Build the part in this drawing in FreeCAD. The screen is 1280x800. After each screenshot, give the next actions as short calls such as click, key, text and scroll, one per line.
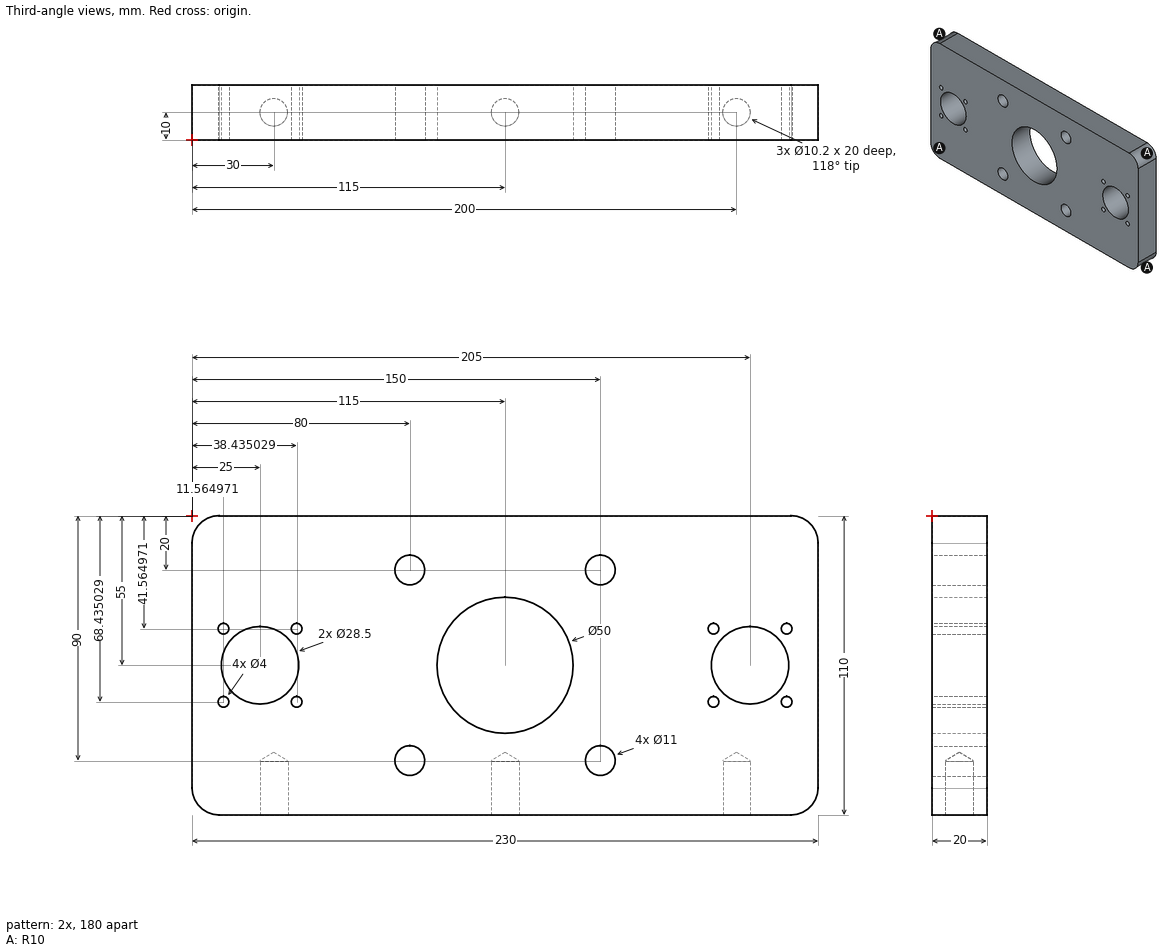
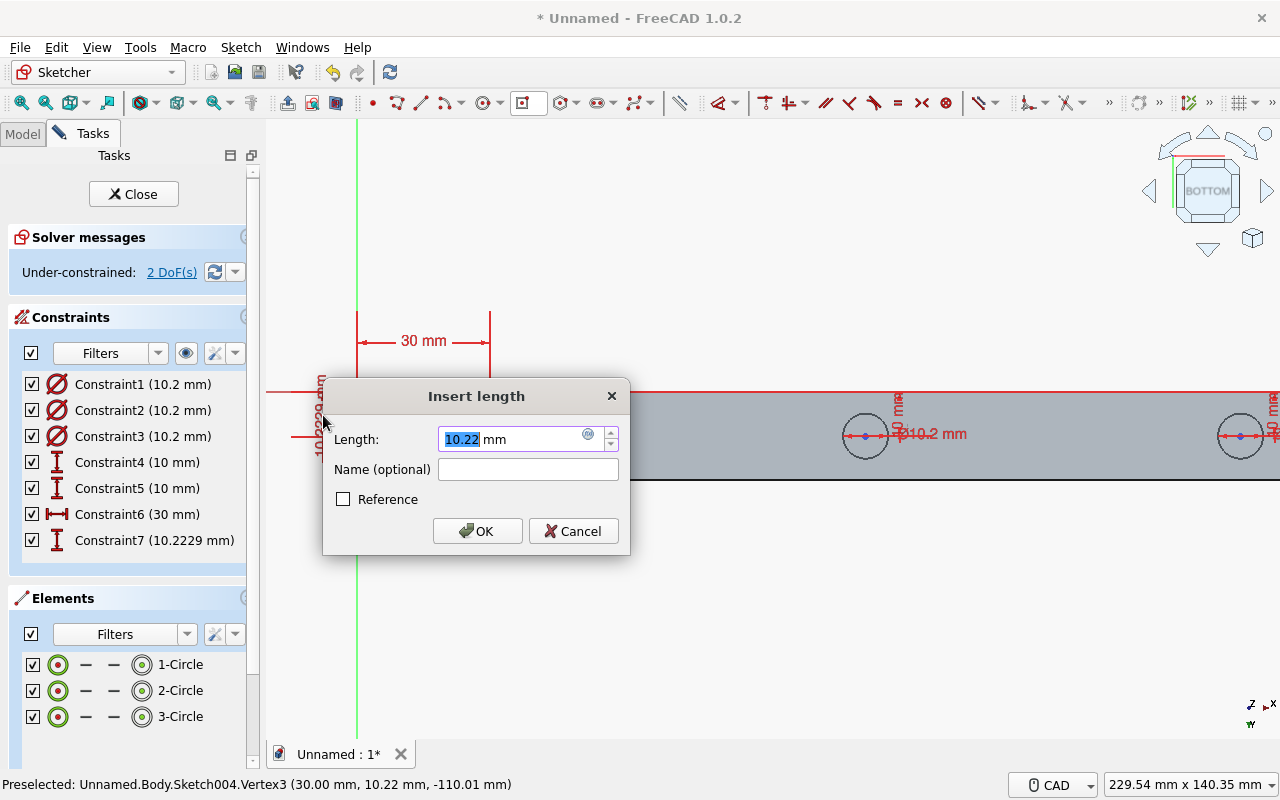
text(10)
key(Return)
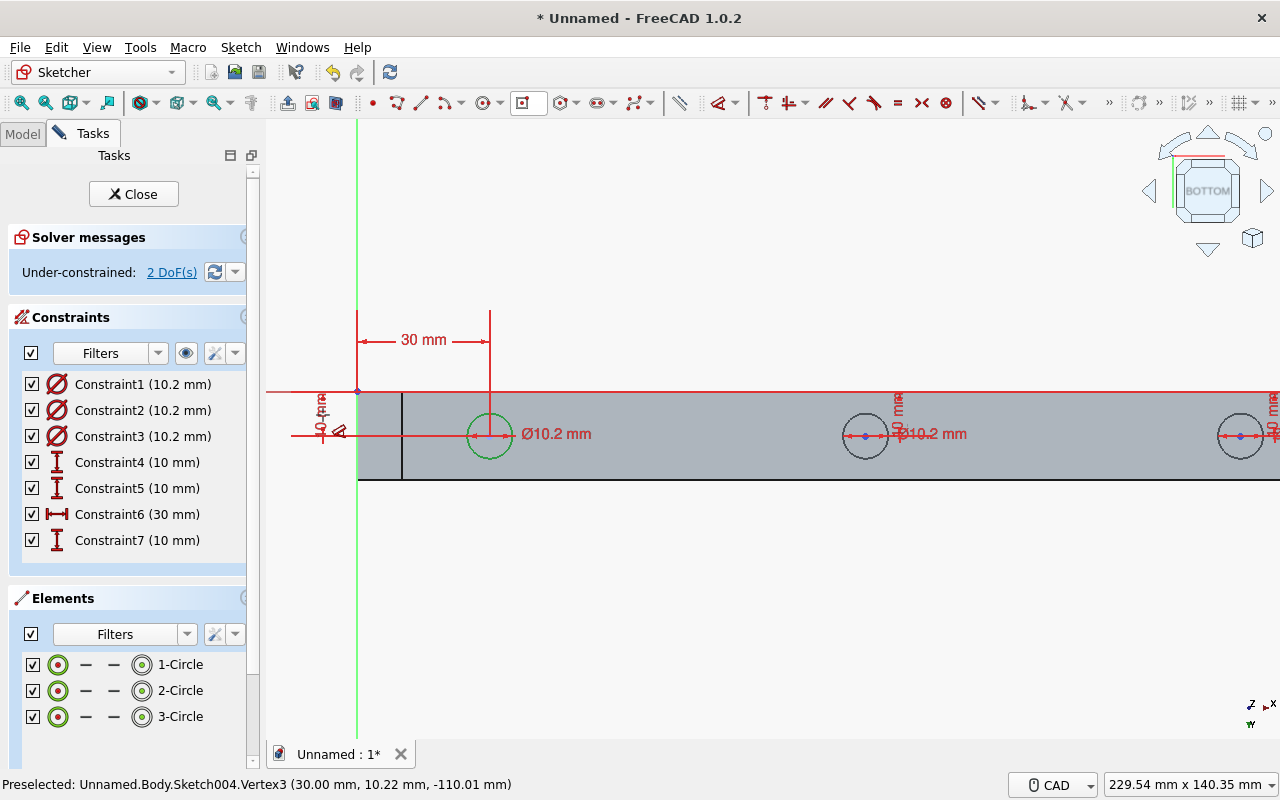
scroll(489, 437, down, 2)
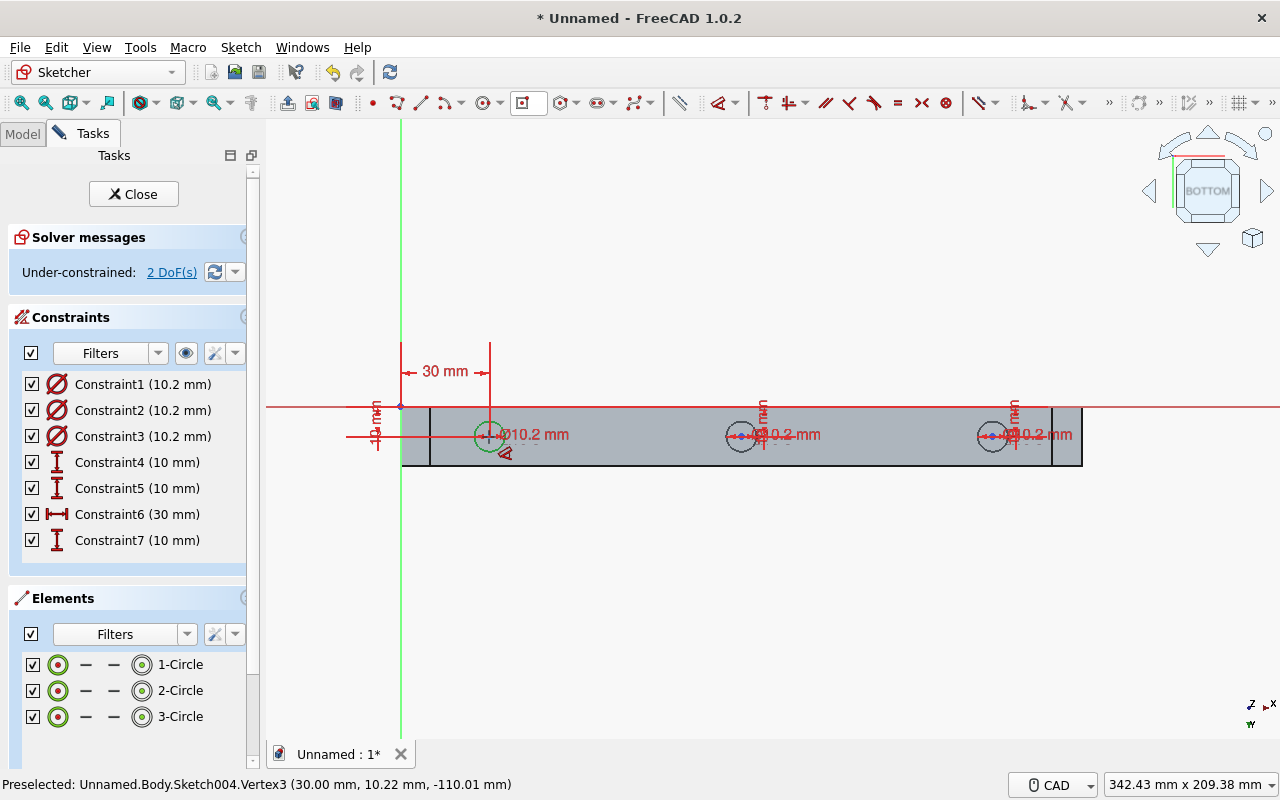
click(993, 437)
click(697, 373)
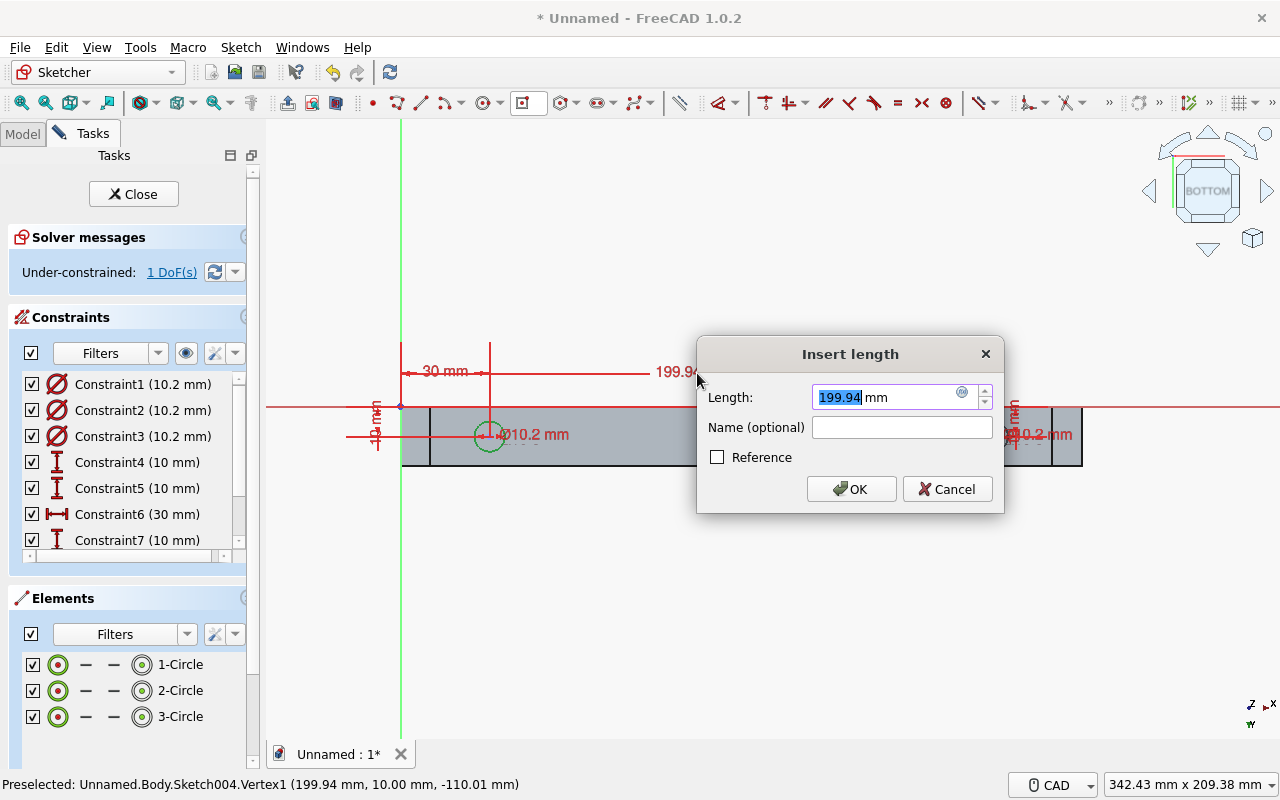
text(200)
key(Return)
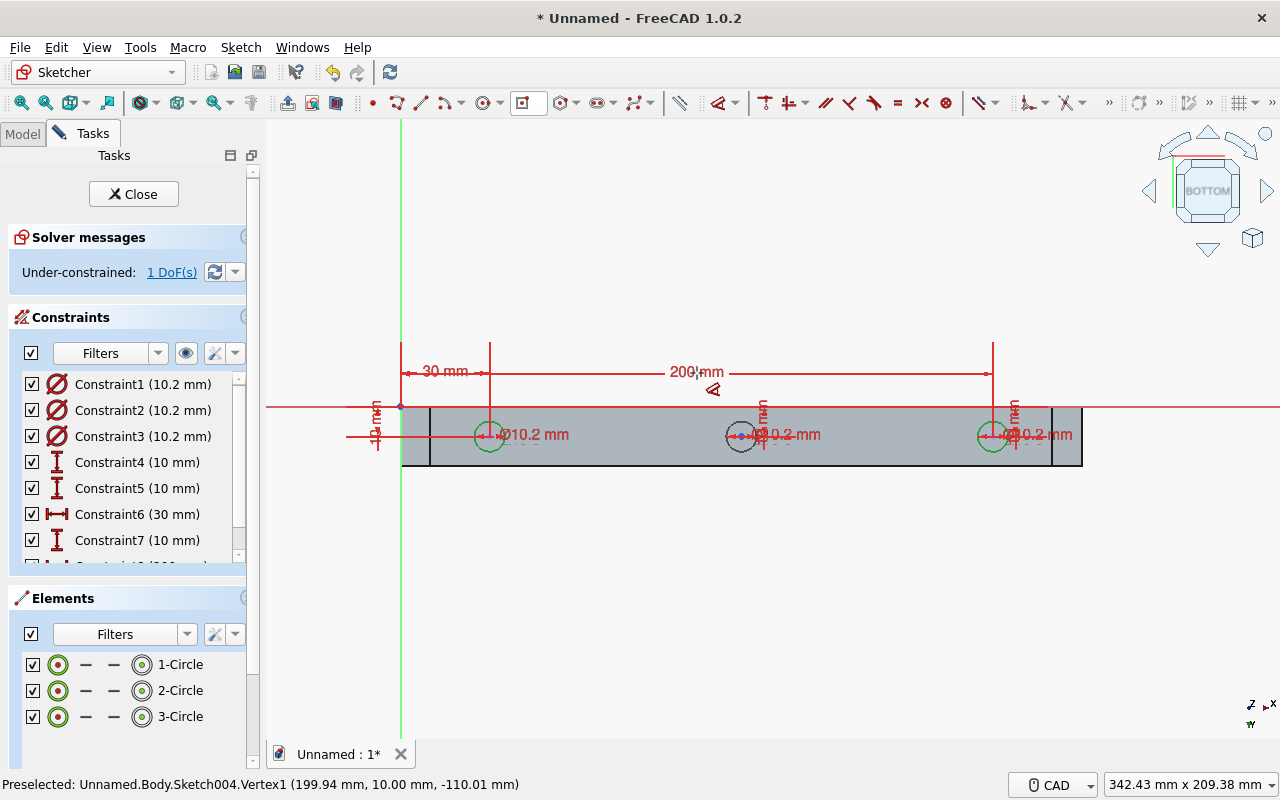
click(742, 437)
click(571, 373)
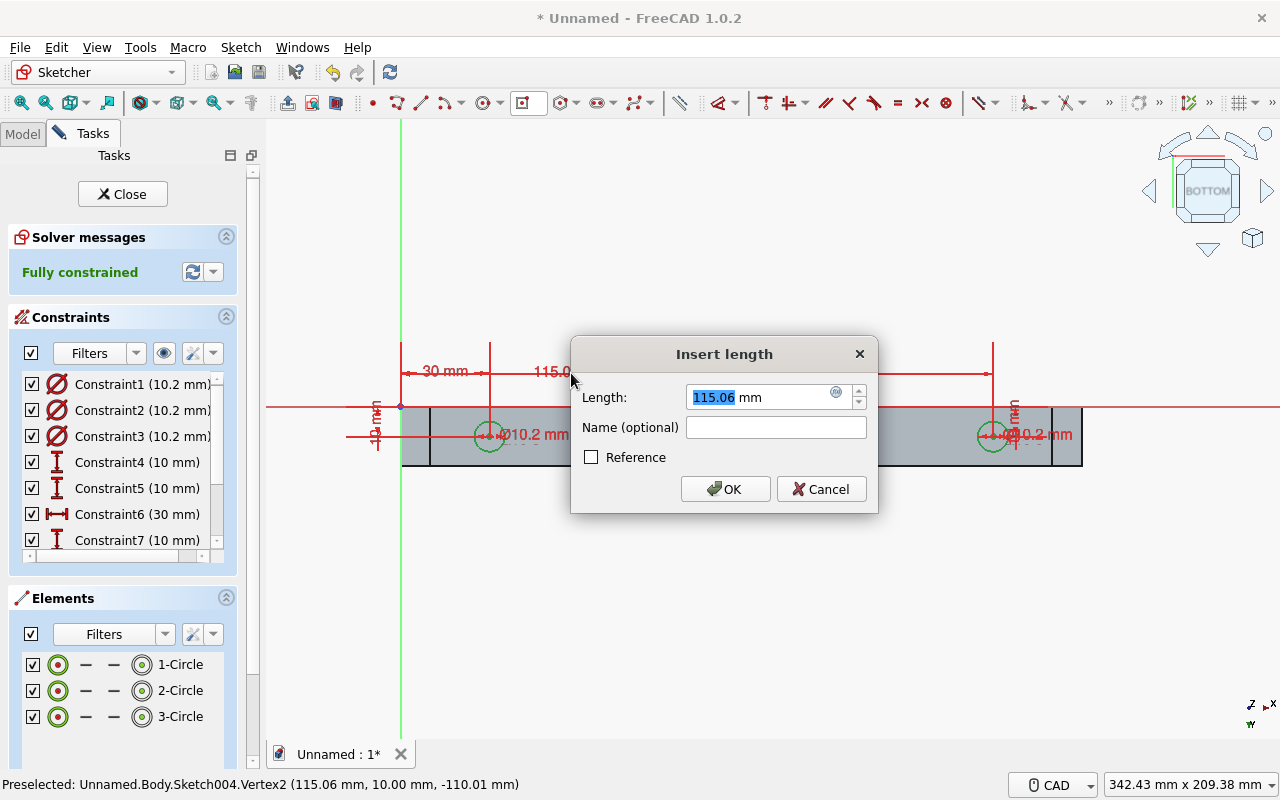
text(115)
key(Return)
key(Escape)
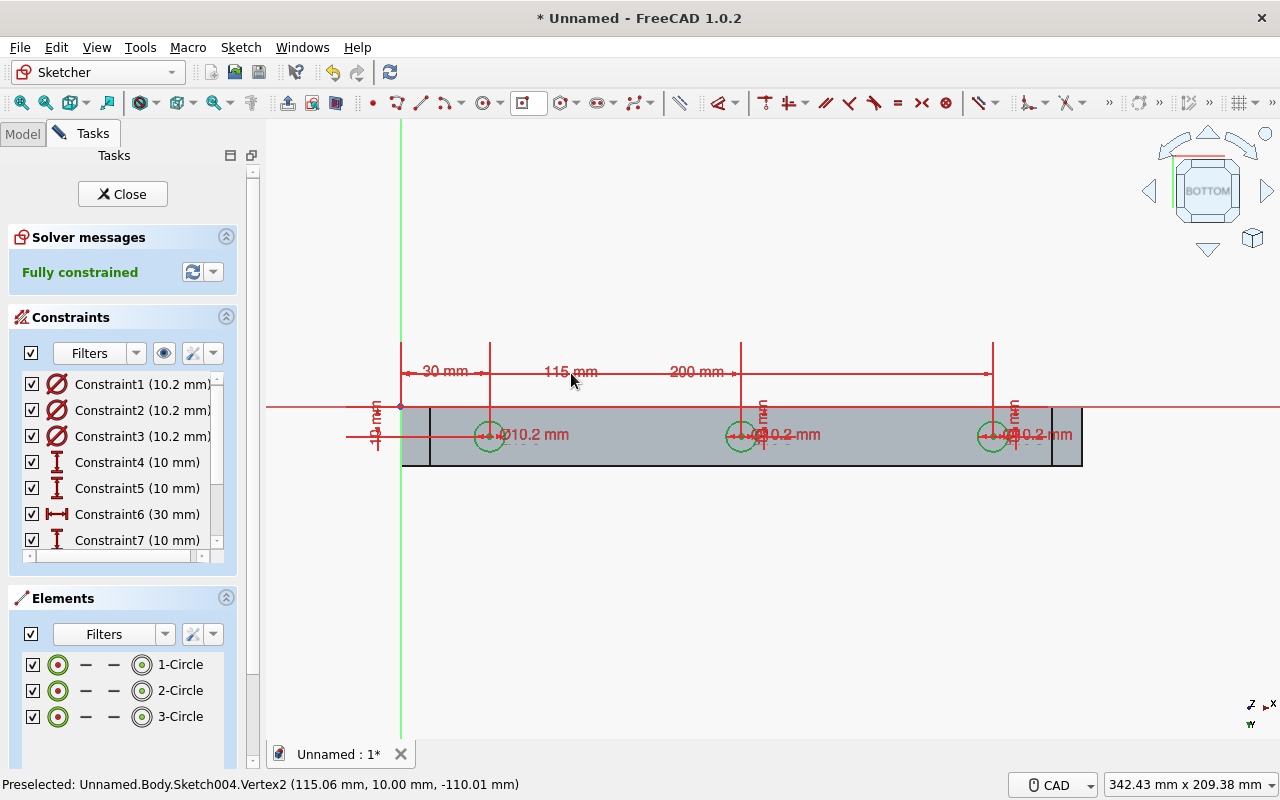
click(123, 194)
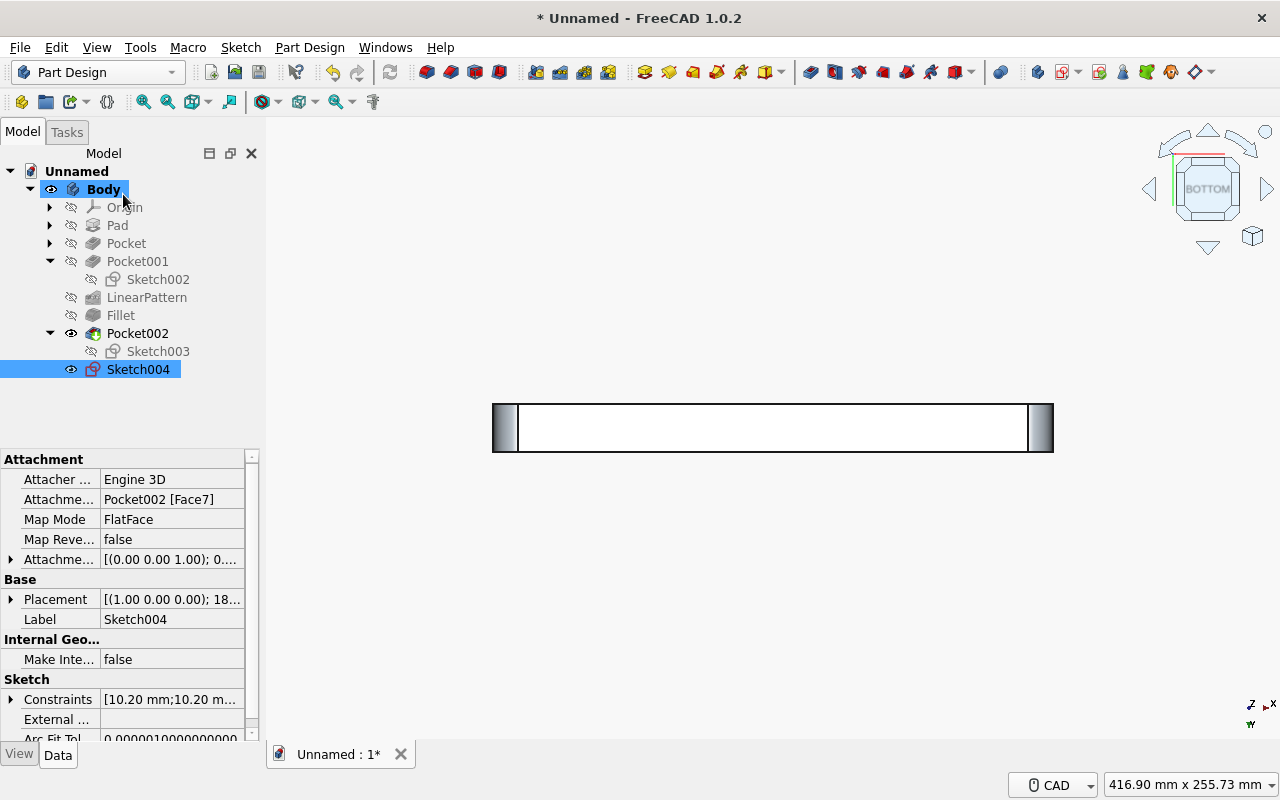
click(836, 72)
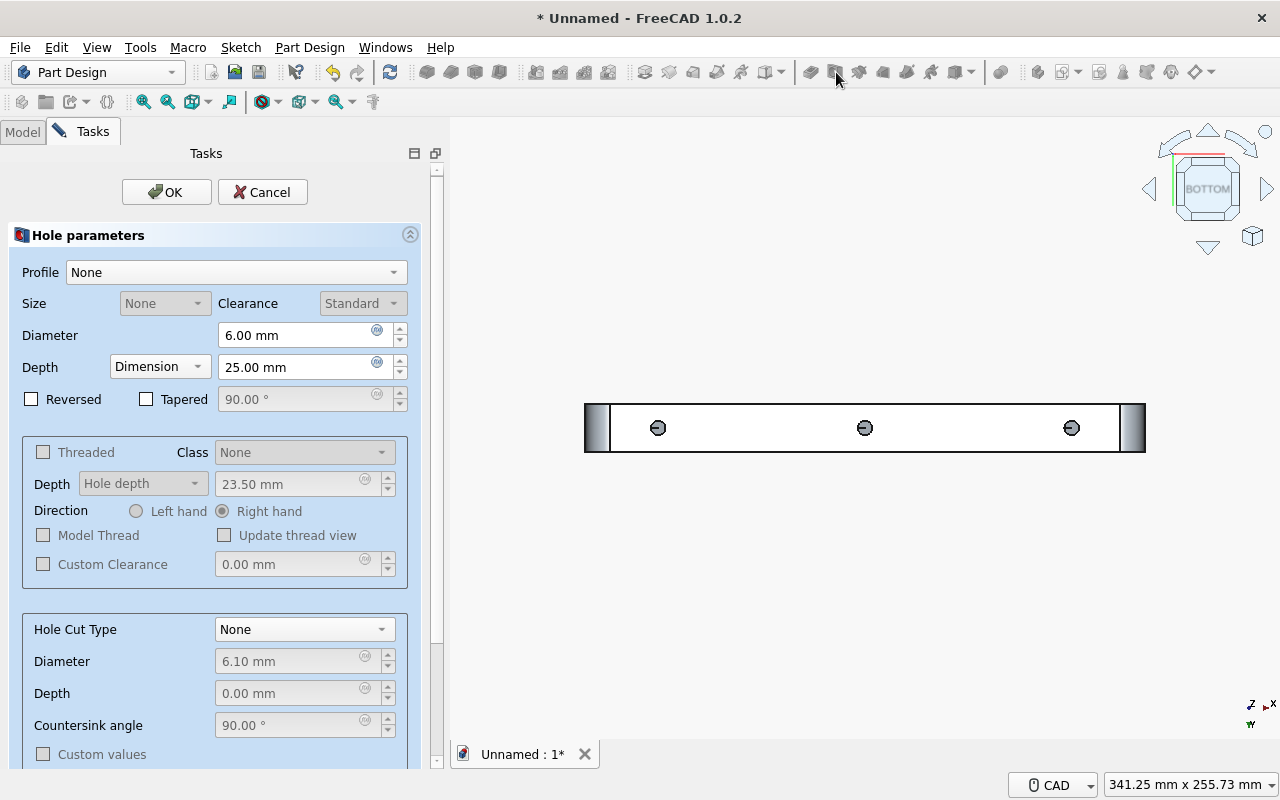
triple_click(305, 335)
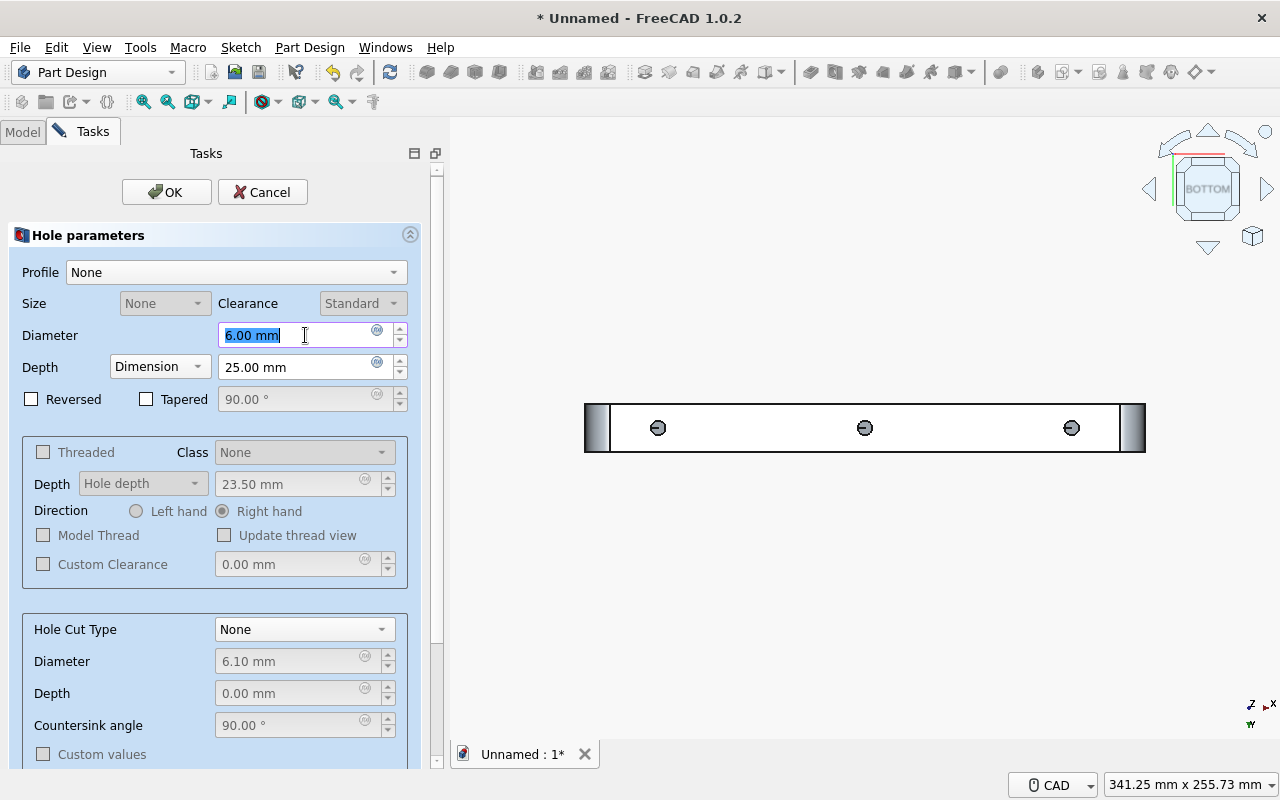
text(10.2)
key(Tab)